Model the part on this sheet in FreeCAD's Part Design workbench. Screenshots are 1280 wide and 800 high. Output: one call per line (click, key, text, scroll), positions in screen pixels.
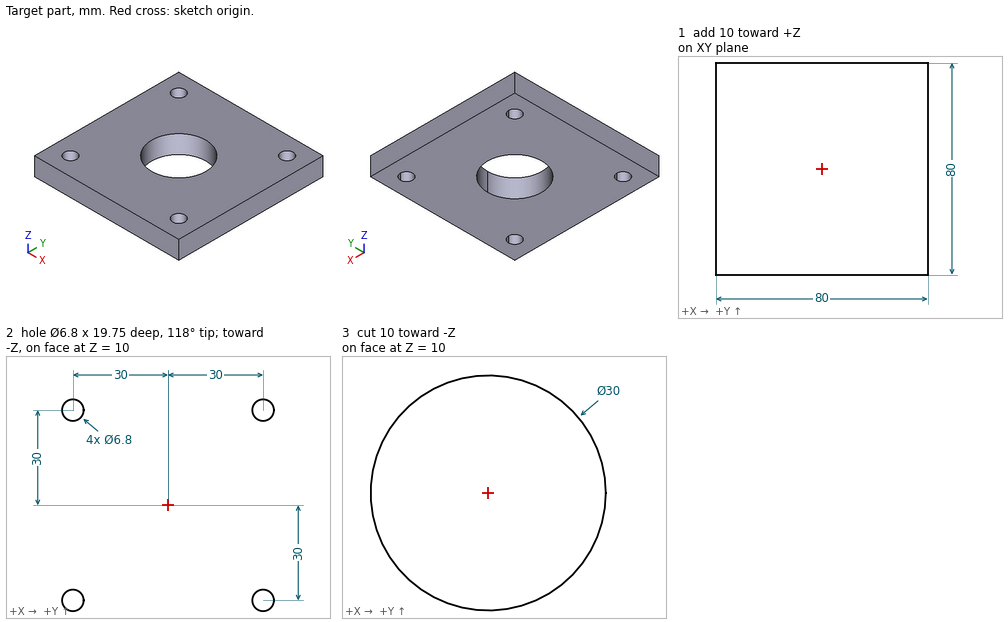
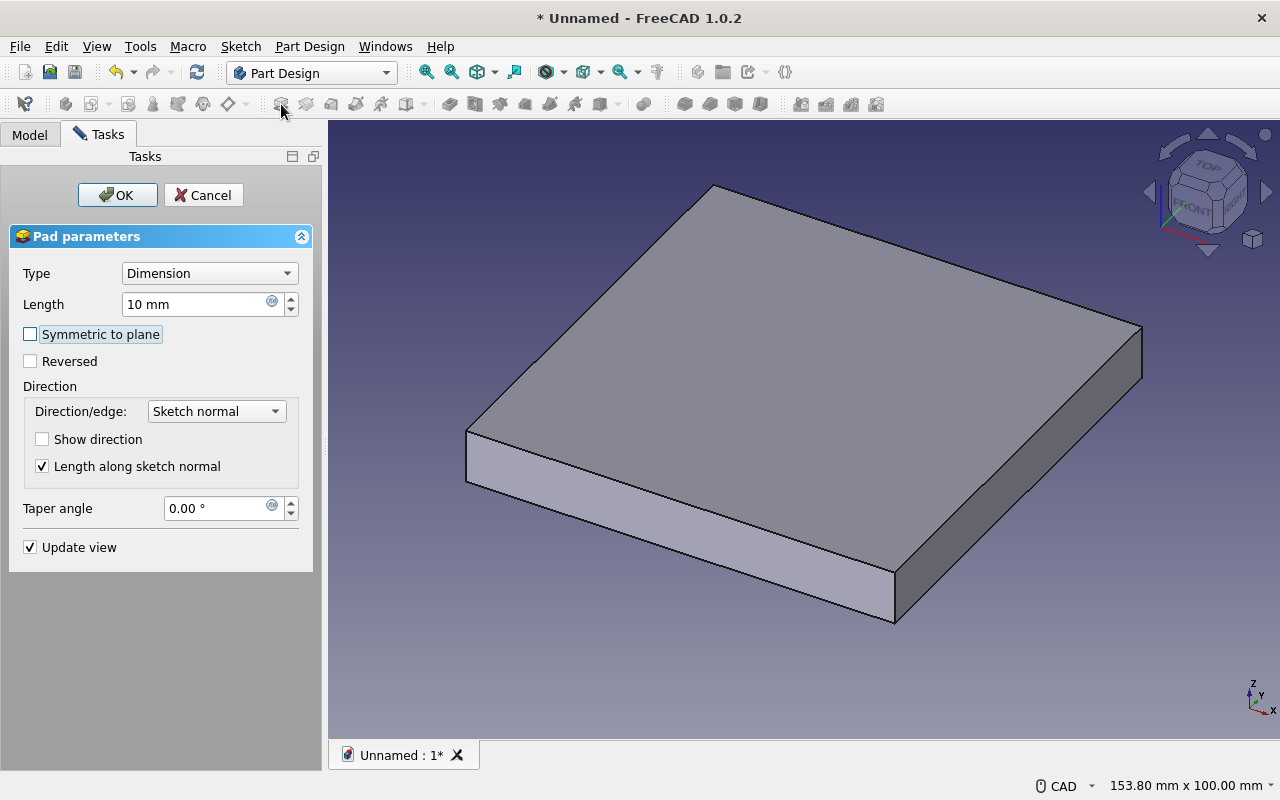
click(118, 195)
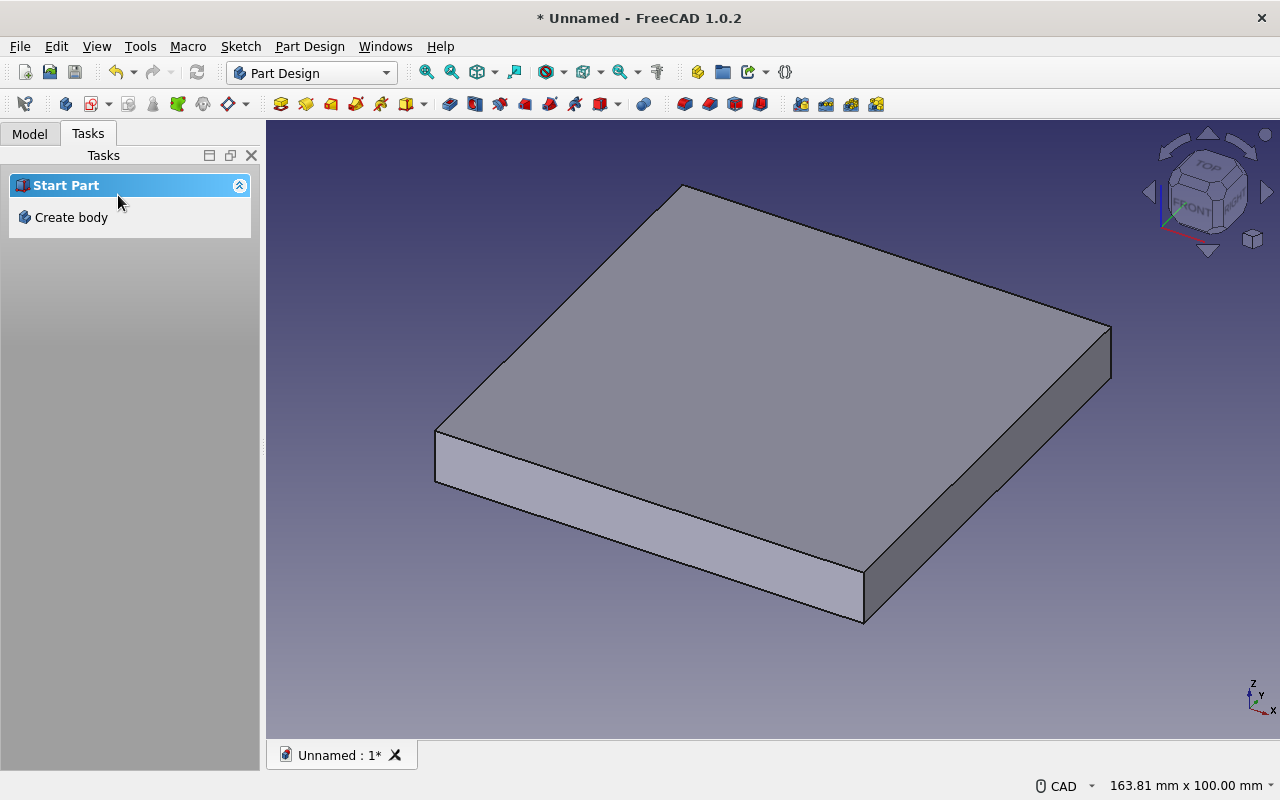
click(773, 378)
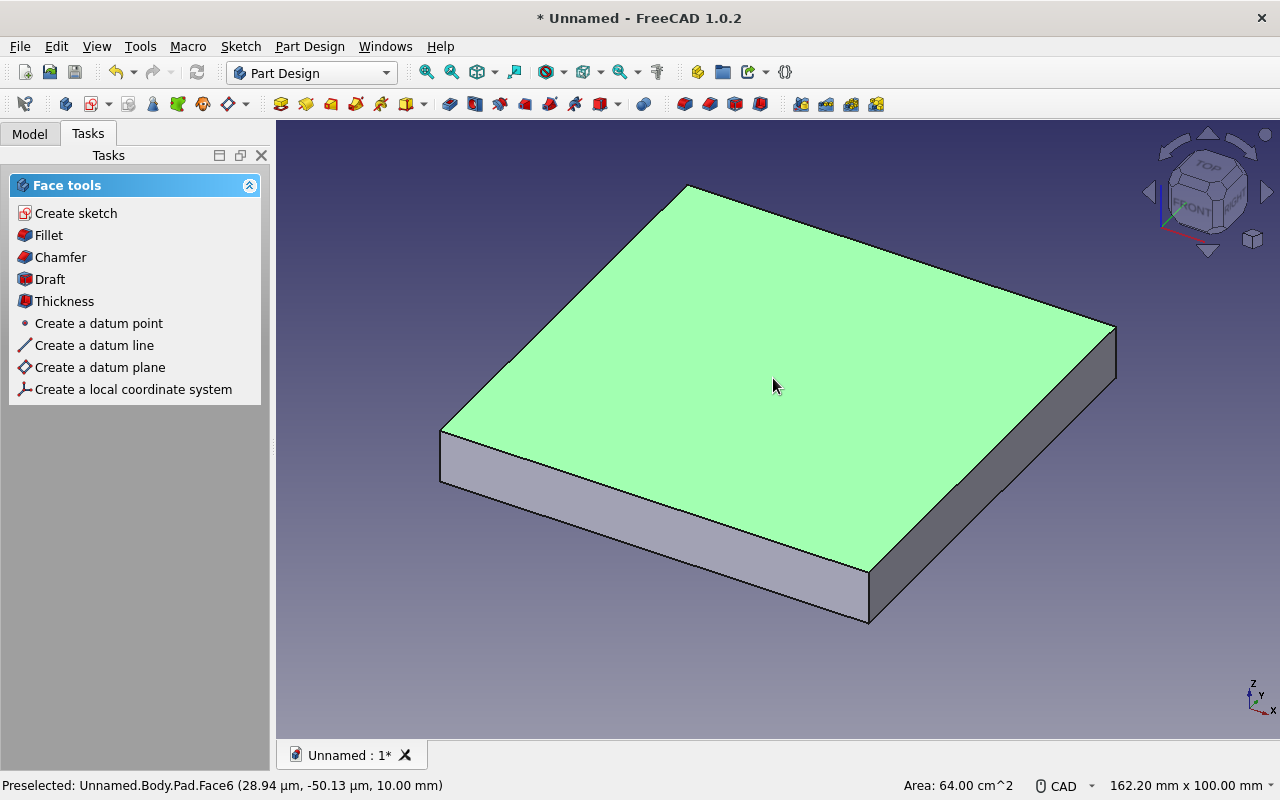
click(90, 104)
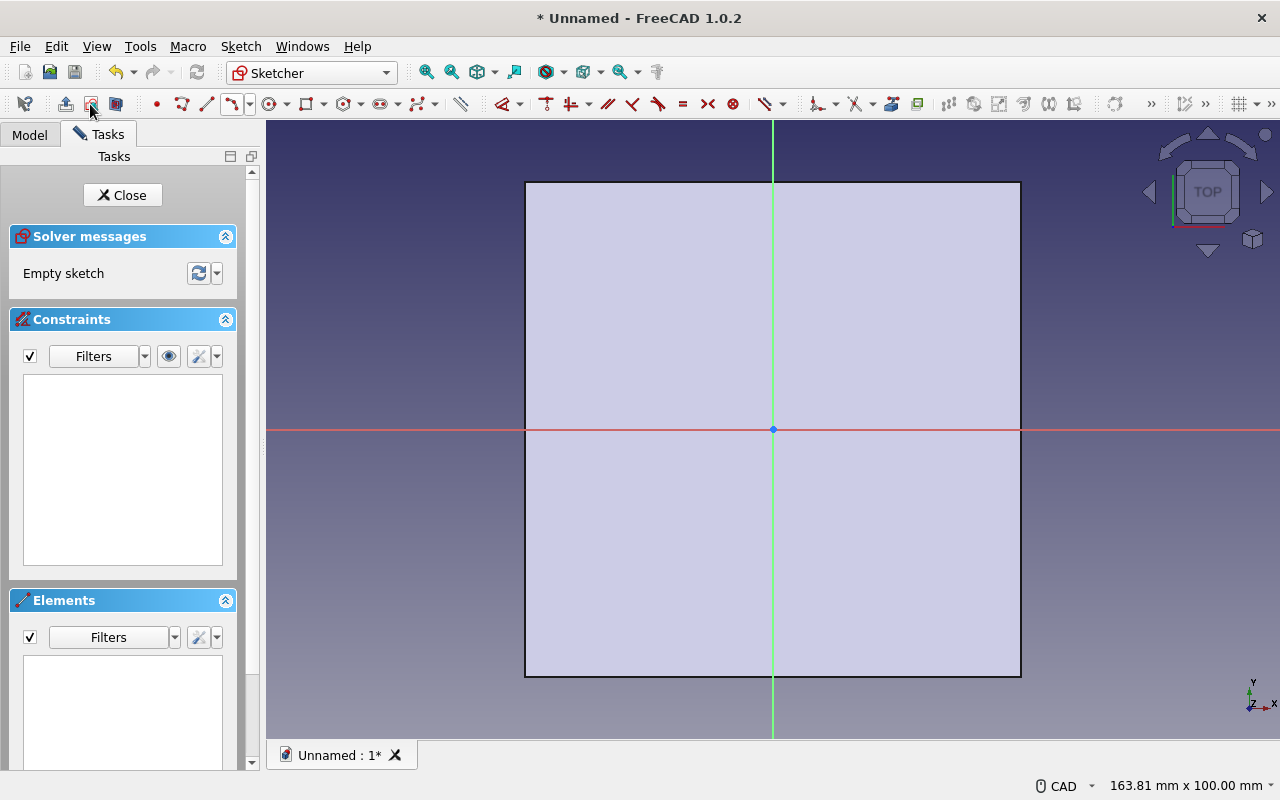
click(268, 104)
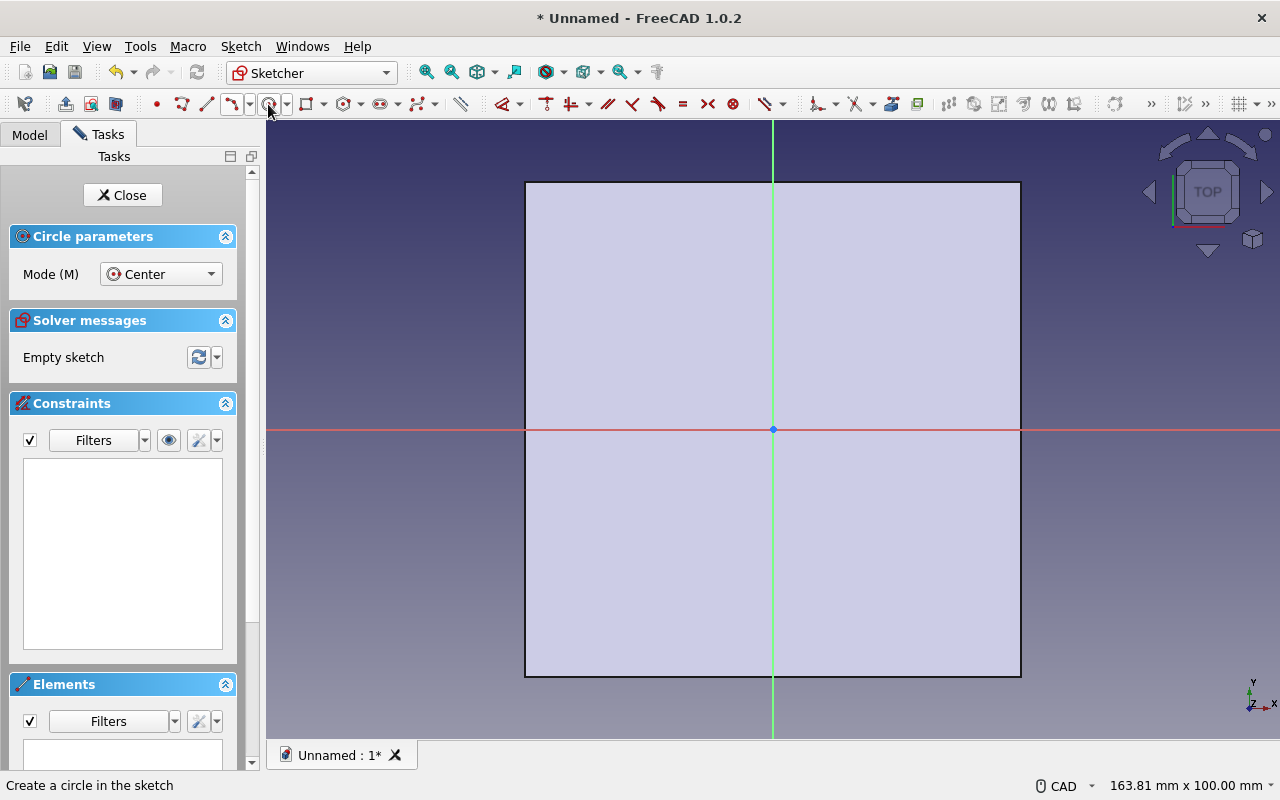
click(587, 244)
move(602, 229)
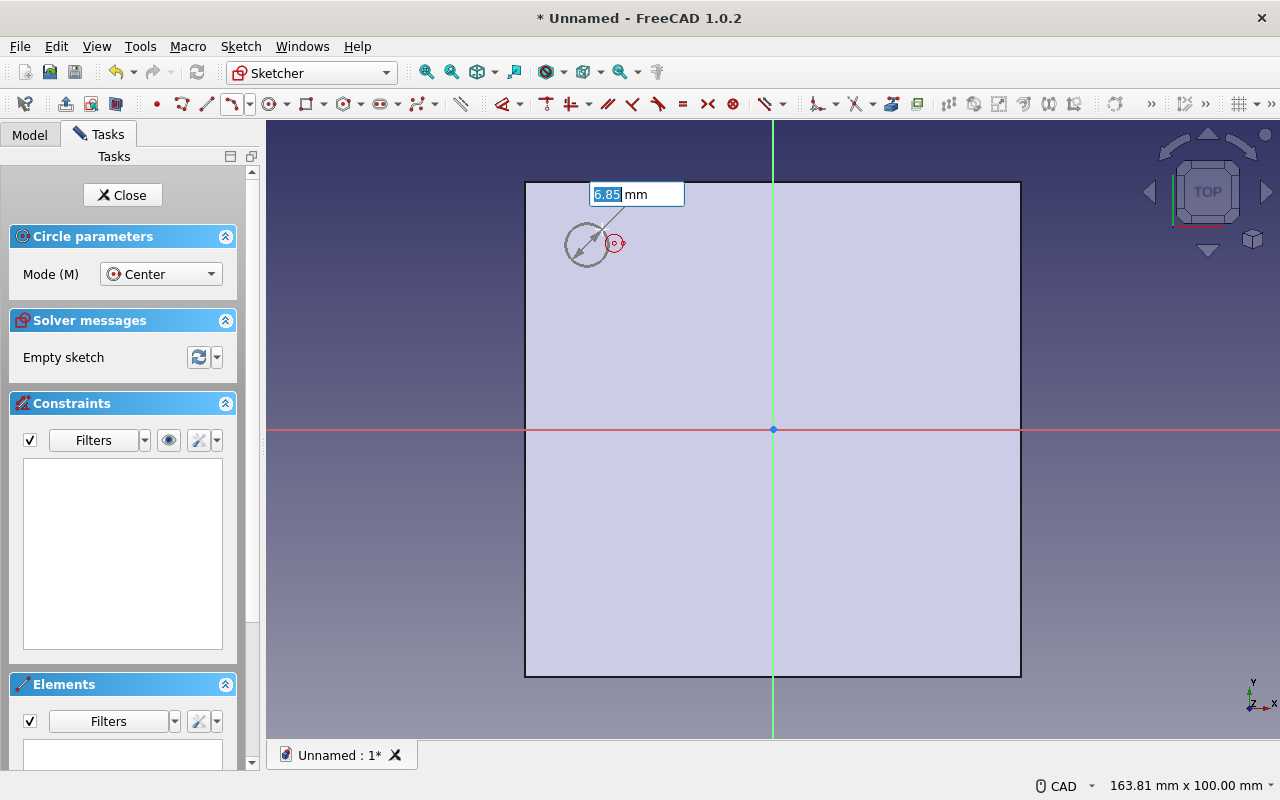
text(6.8)
key(Return)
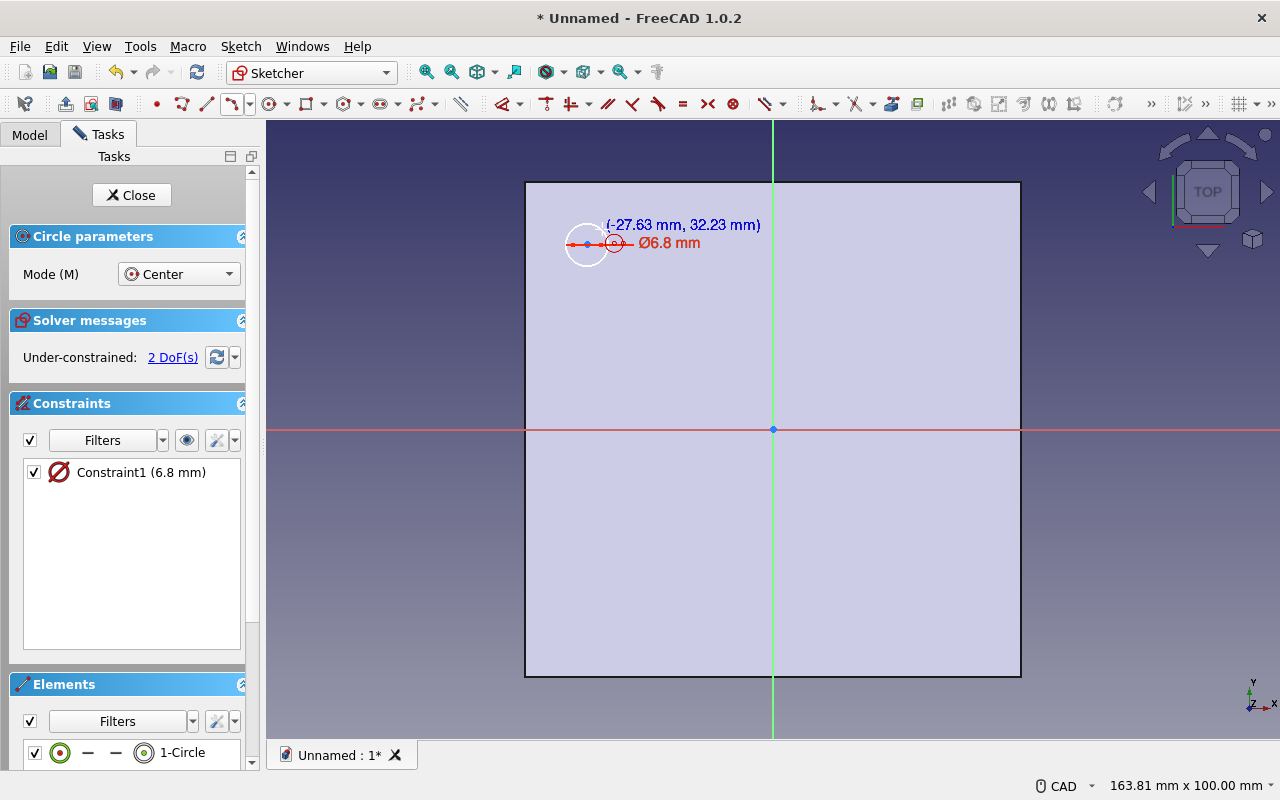
click(959, 244)
move(974, 229)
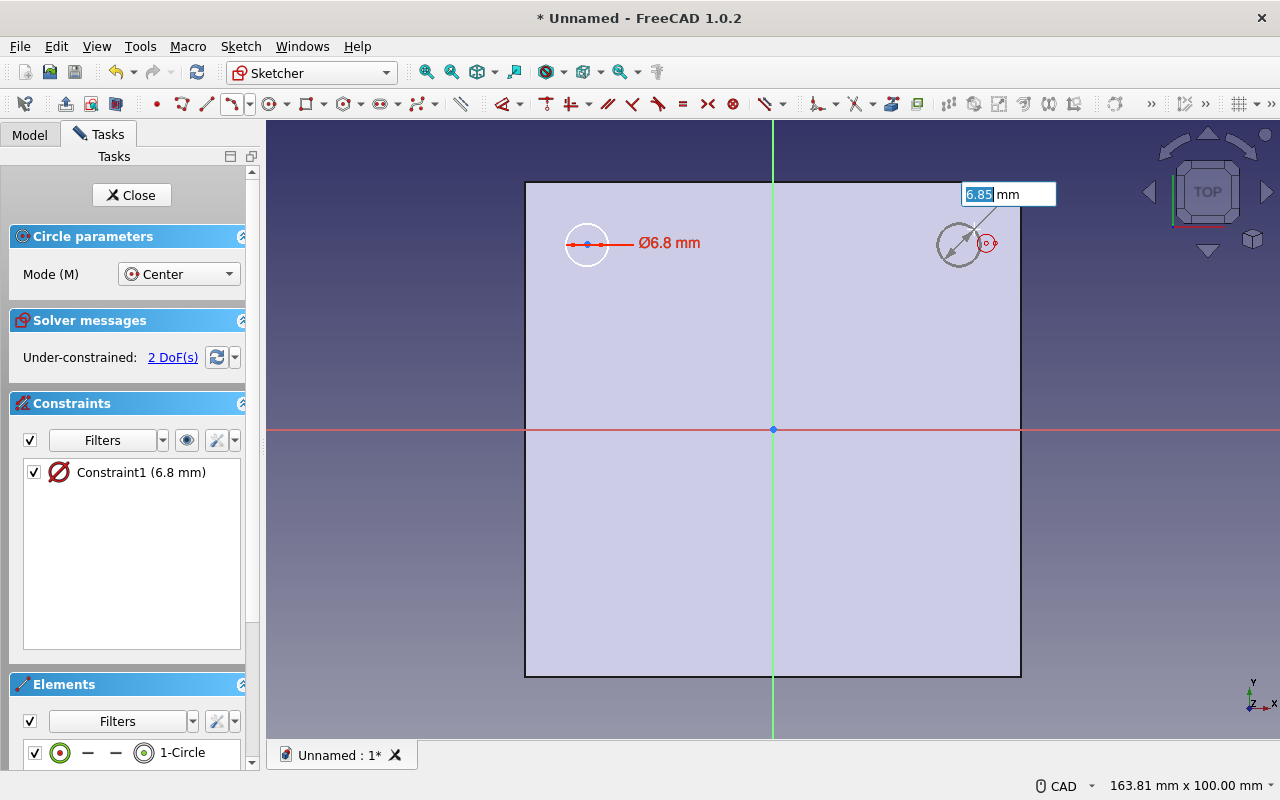
text(6.8)
key(Return)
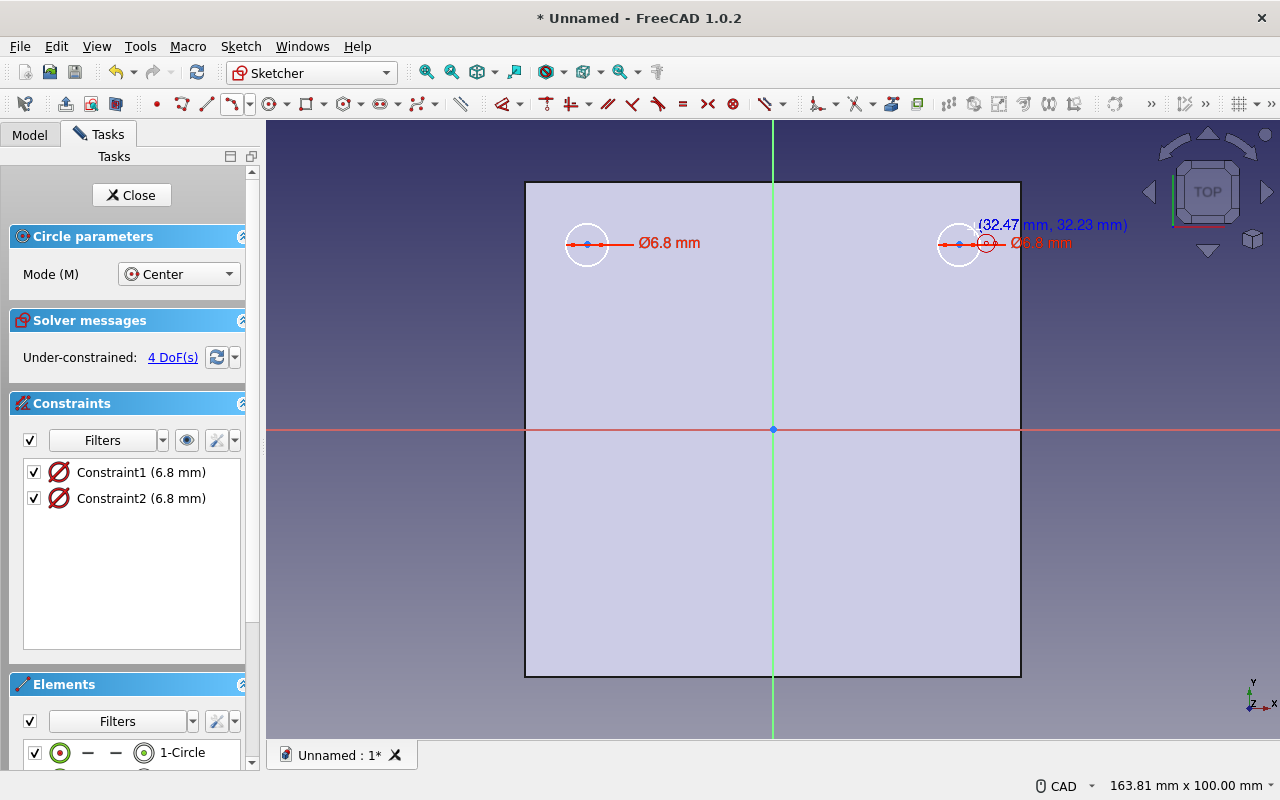
click(959, 615)
move(974, 600)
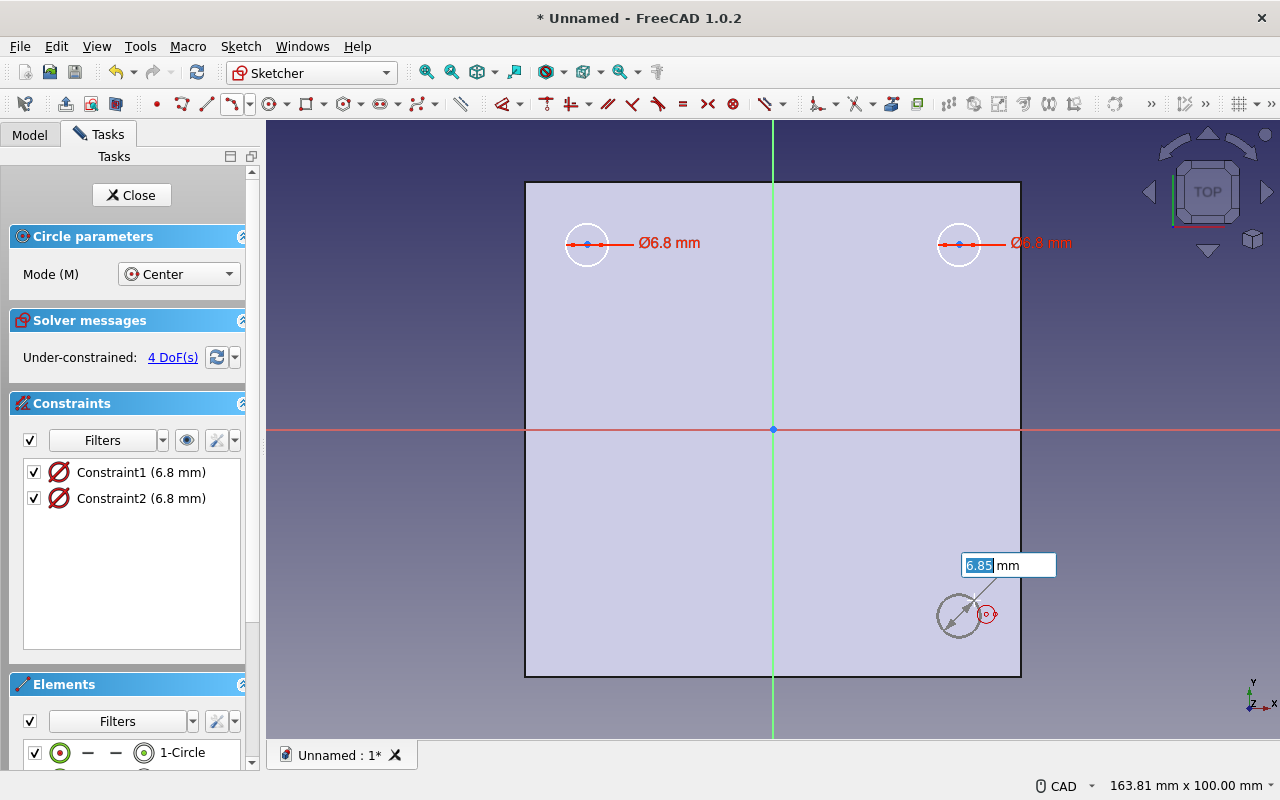
text(6.8)
key(Return)